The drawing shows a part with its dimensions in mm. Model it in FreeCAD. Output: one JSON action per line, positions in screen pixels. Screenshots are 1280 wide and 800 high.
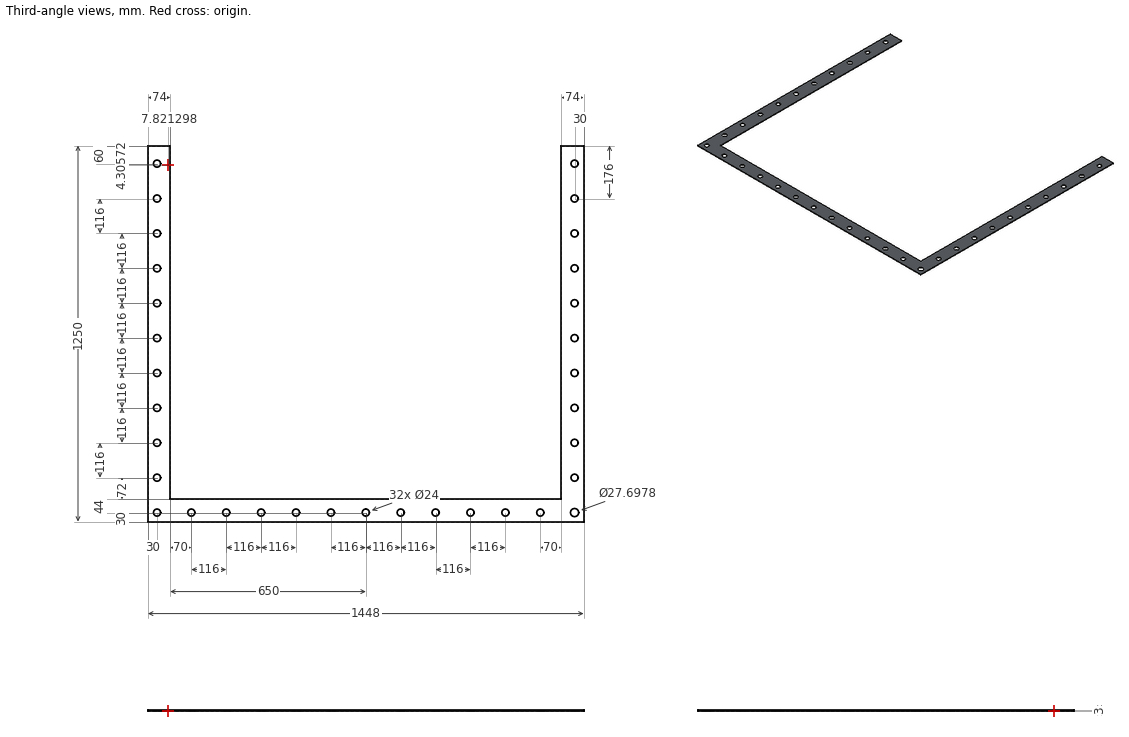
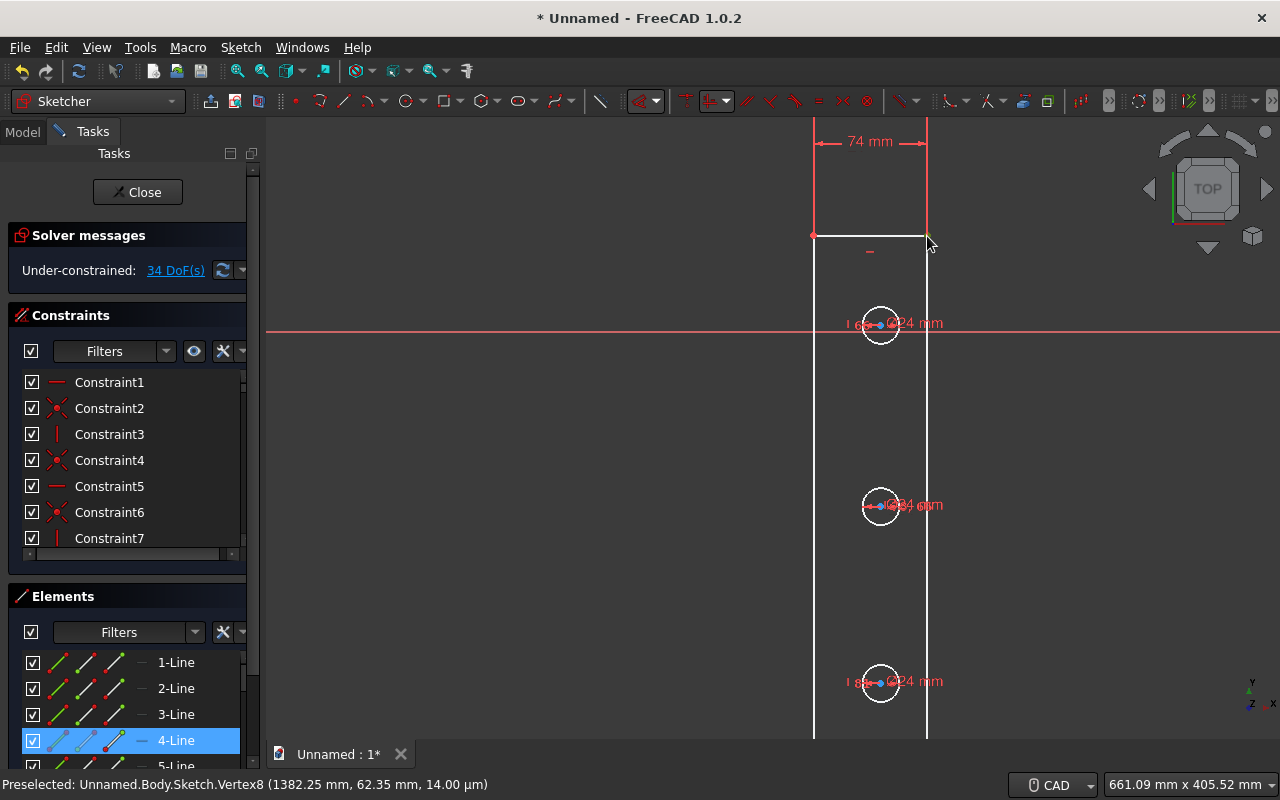
{"action": "left_click", "coordinate": [881, 507]}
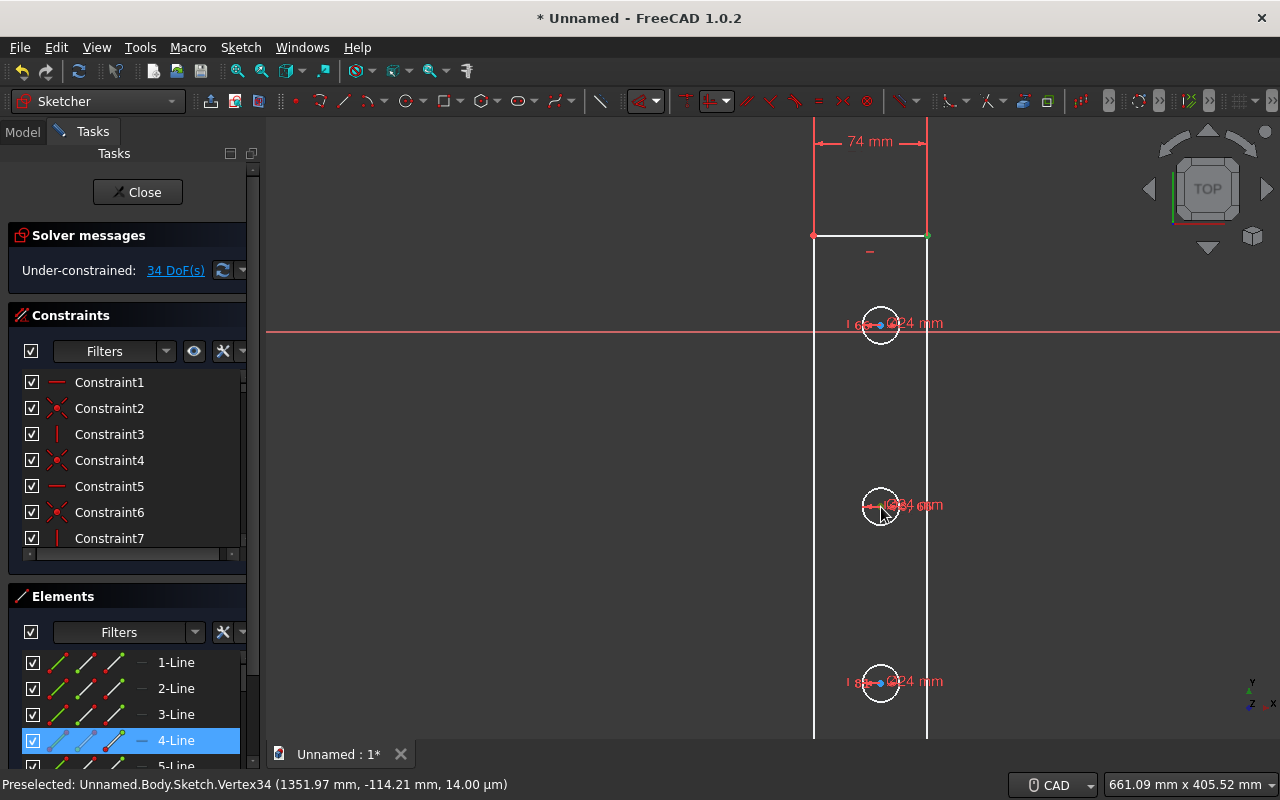
{"action": "key", "text": "l"}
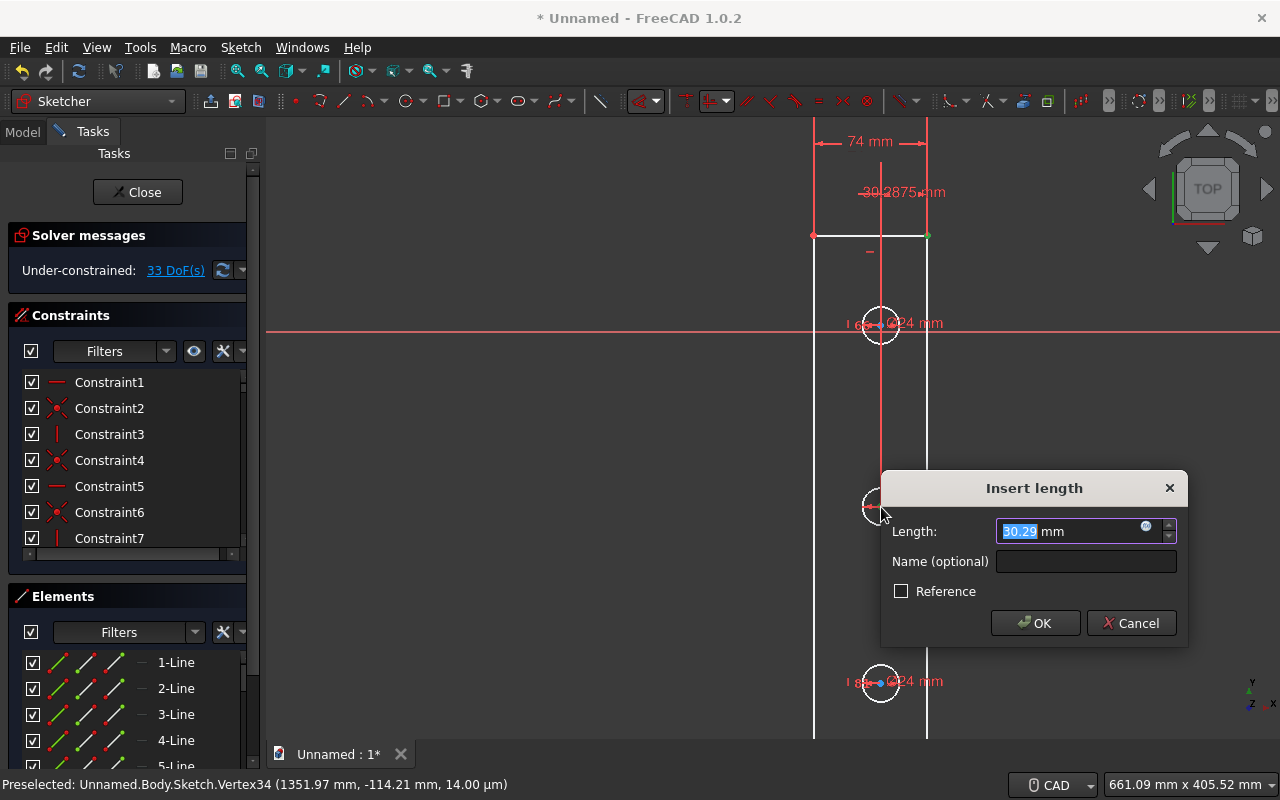
{"action": "type", "text": "30"}
{"action": "key", "text": "Return"}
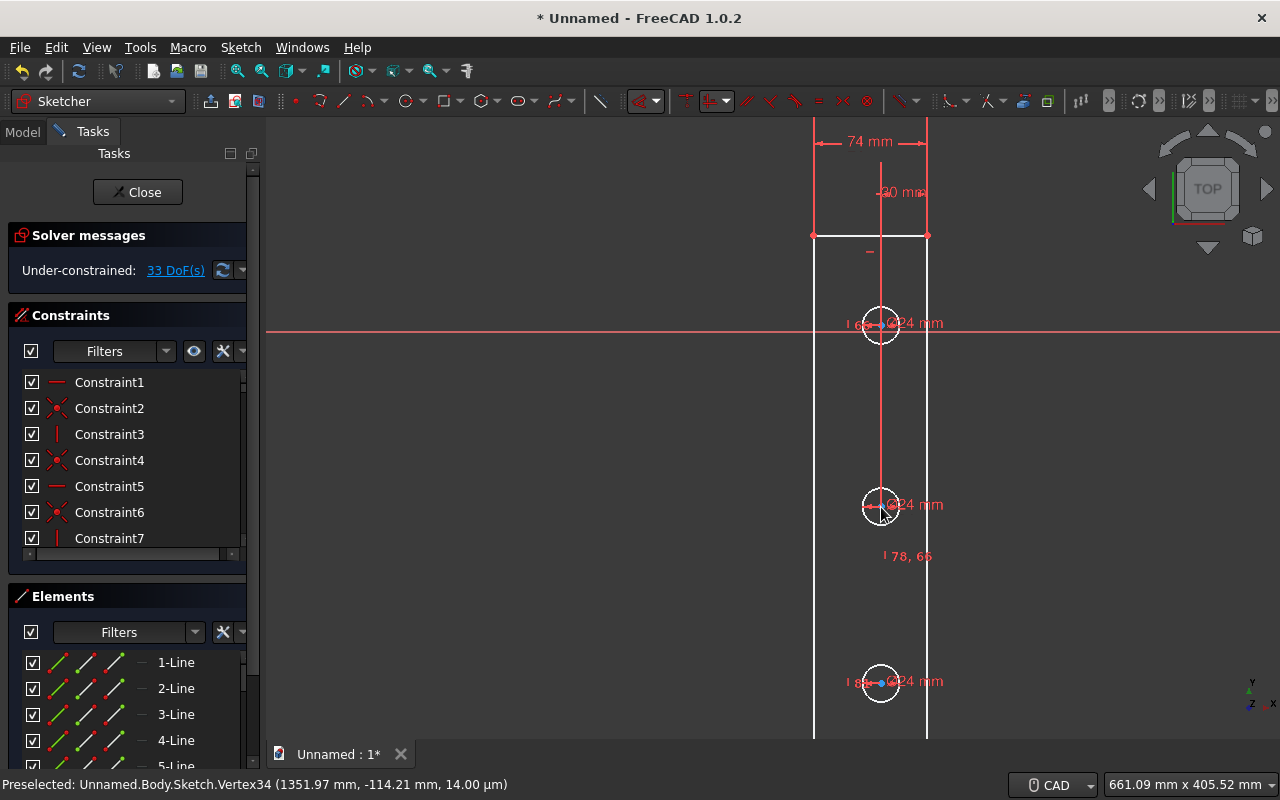
{"action": "left_click", "coordinate": [927, 236]}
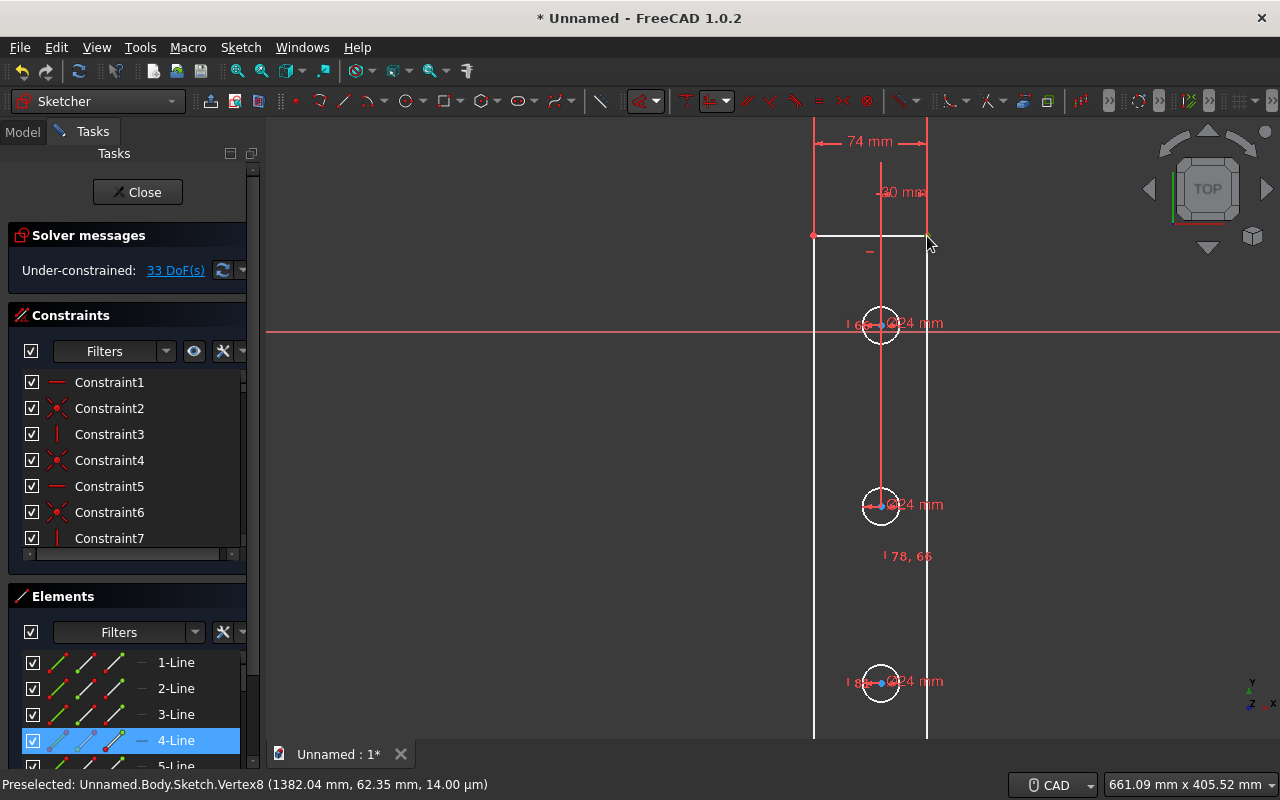
{"action": "left_click", "coordinate": [881, 325]}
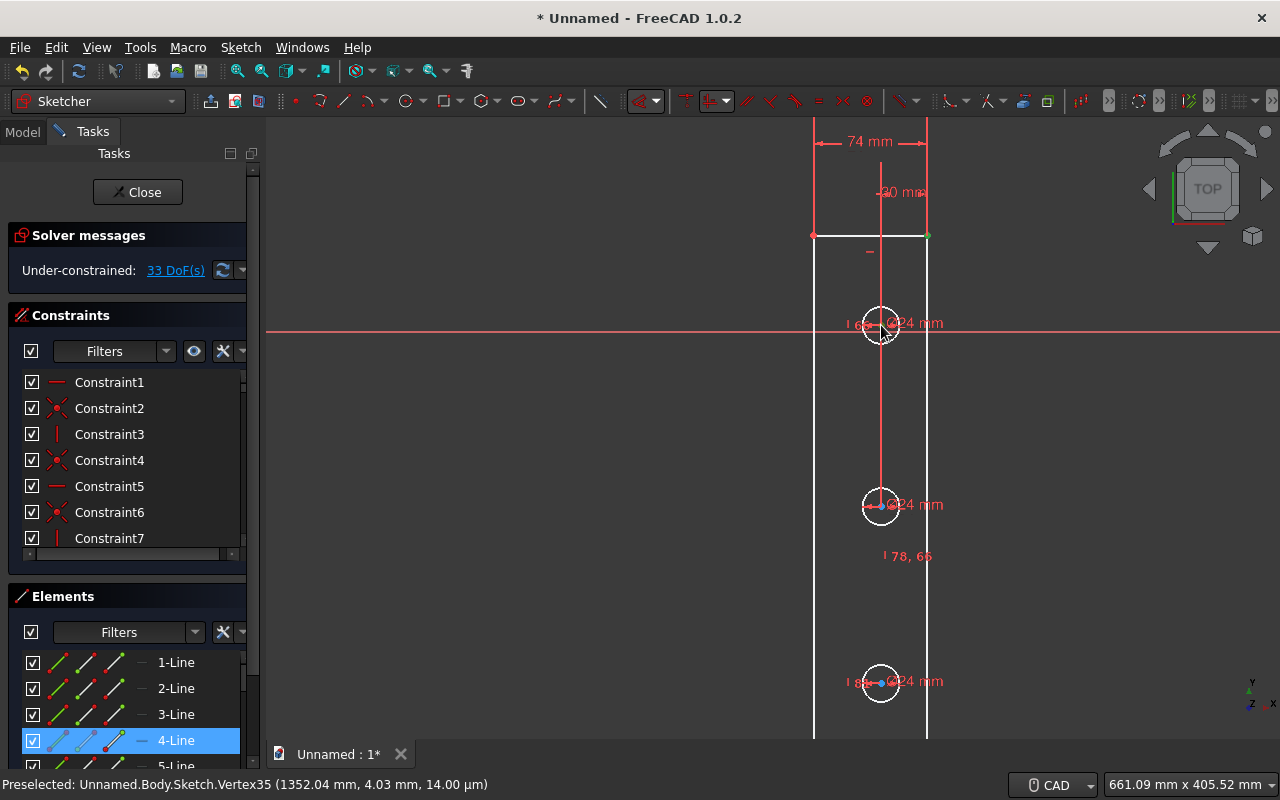
{"action": "key", "text": "i"}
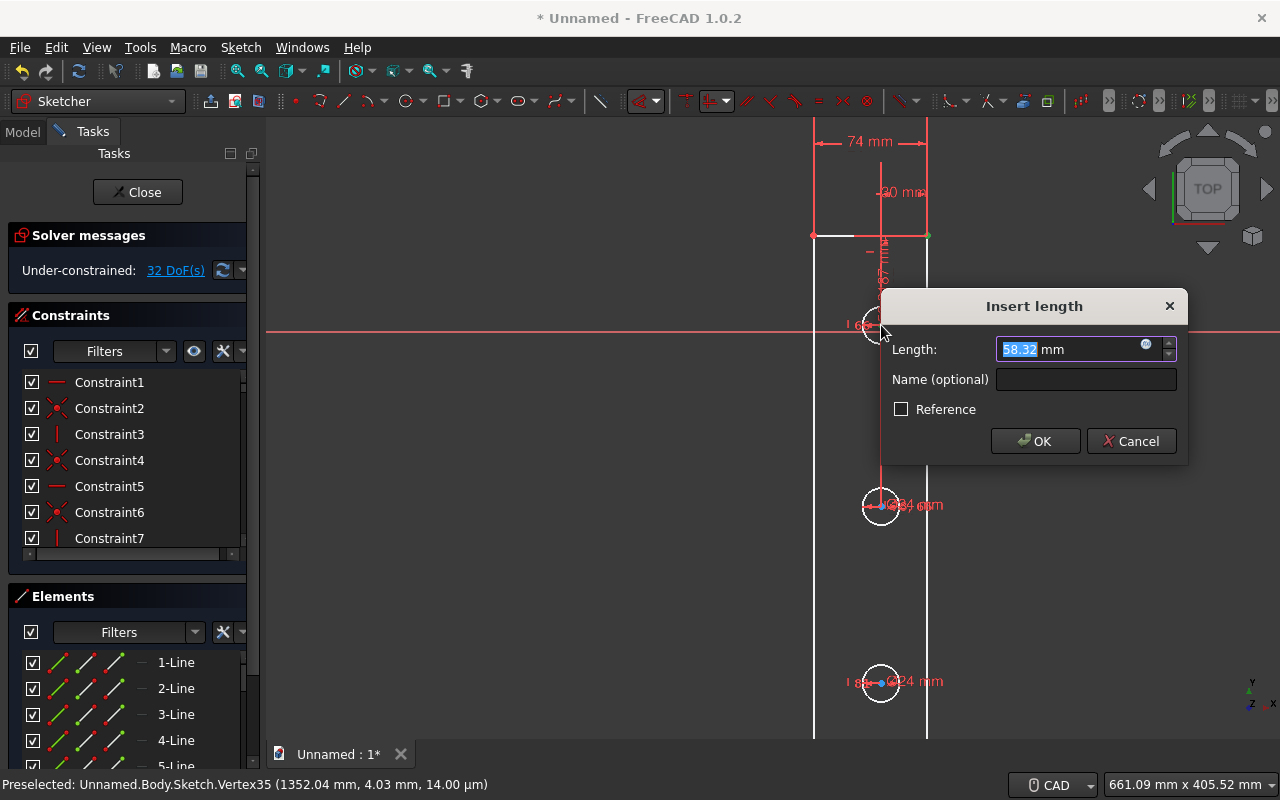
{"action": "type", "text": "60"}
{"action": "key", "text": "Return"}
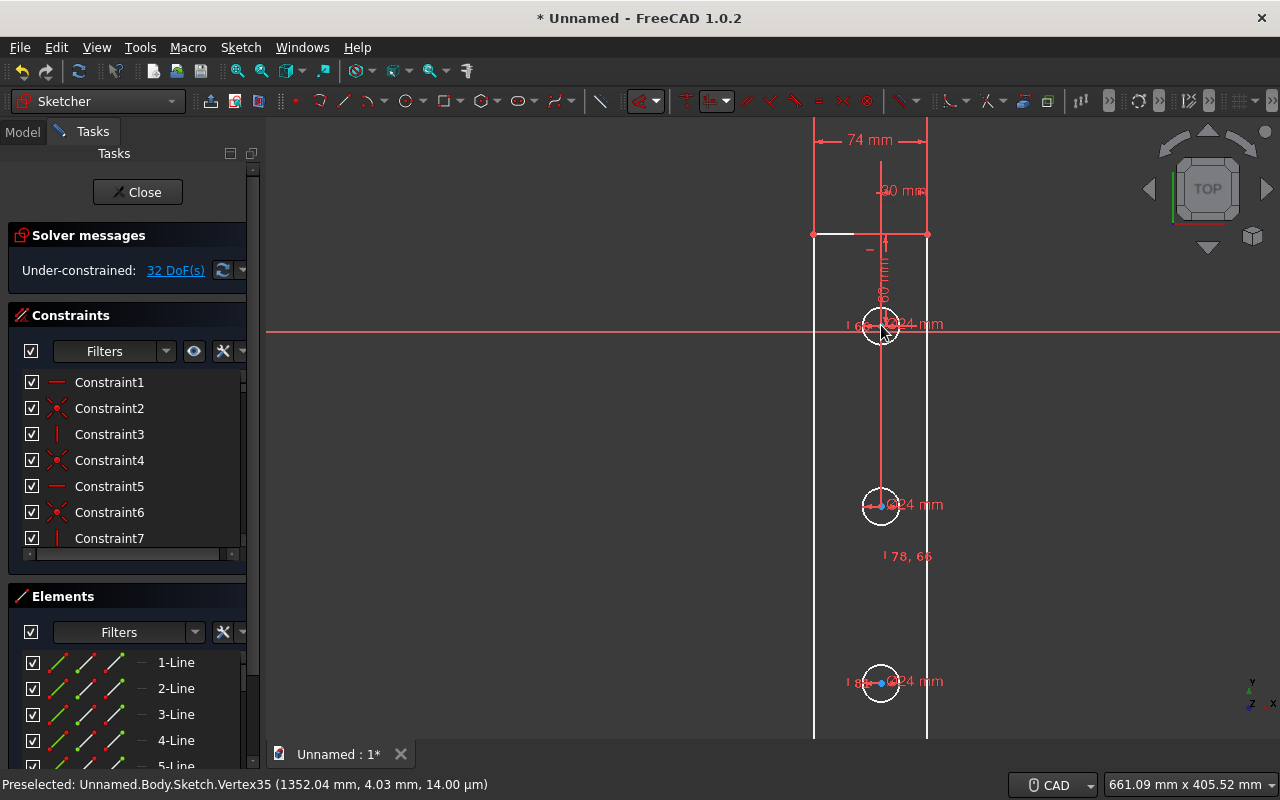
{"action": "scroll", "coordinate": [929, 235], "scroll_direction": "down", "scroll_amount": 8}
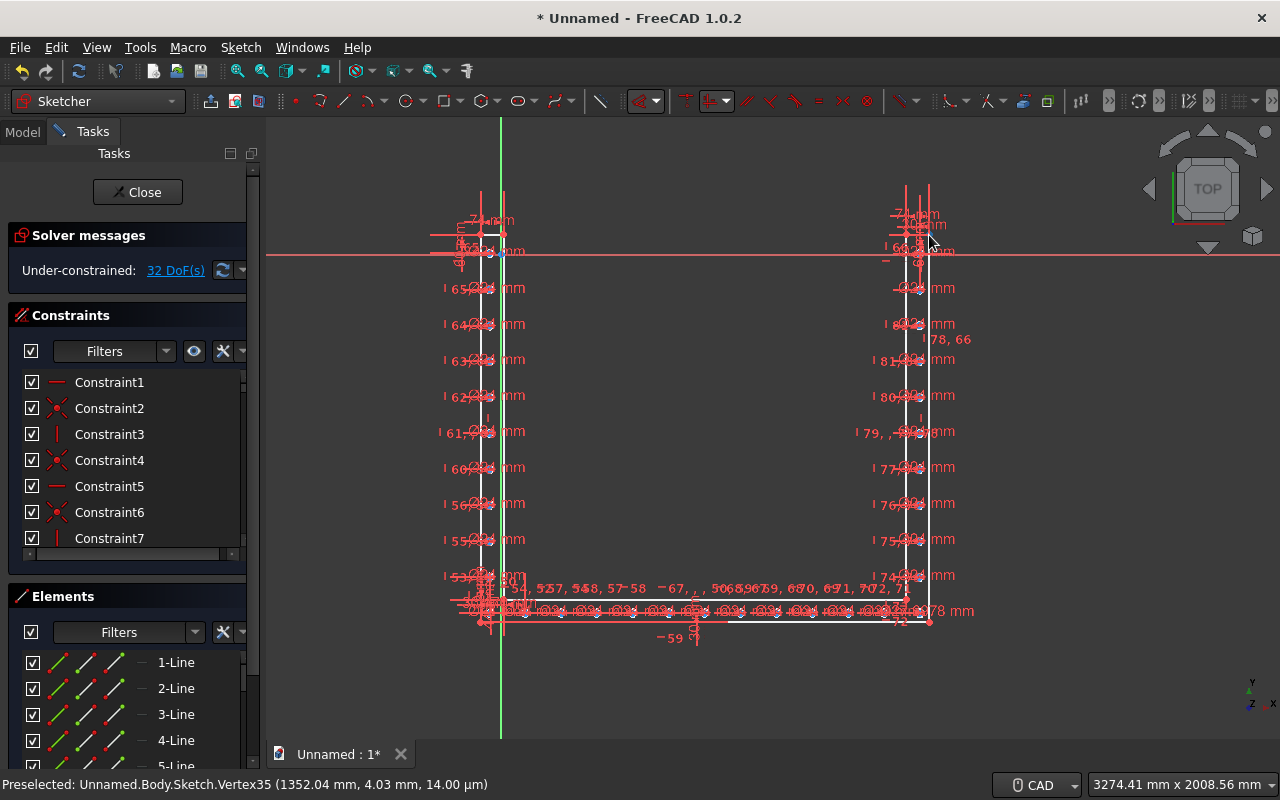
{"action": "scroll", "coordinate": [906, 600], "scroll_direction": "up", "scroll_amount": 4}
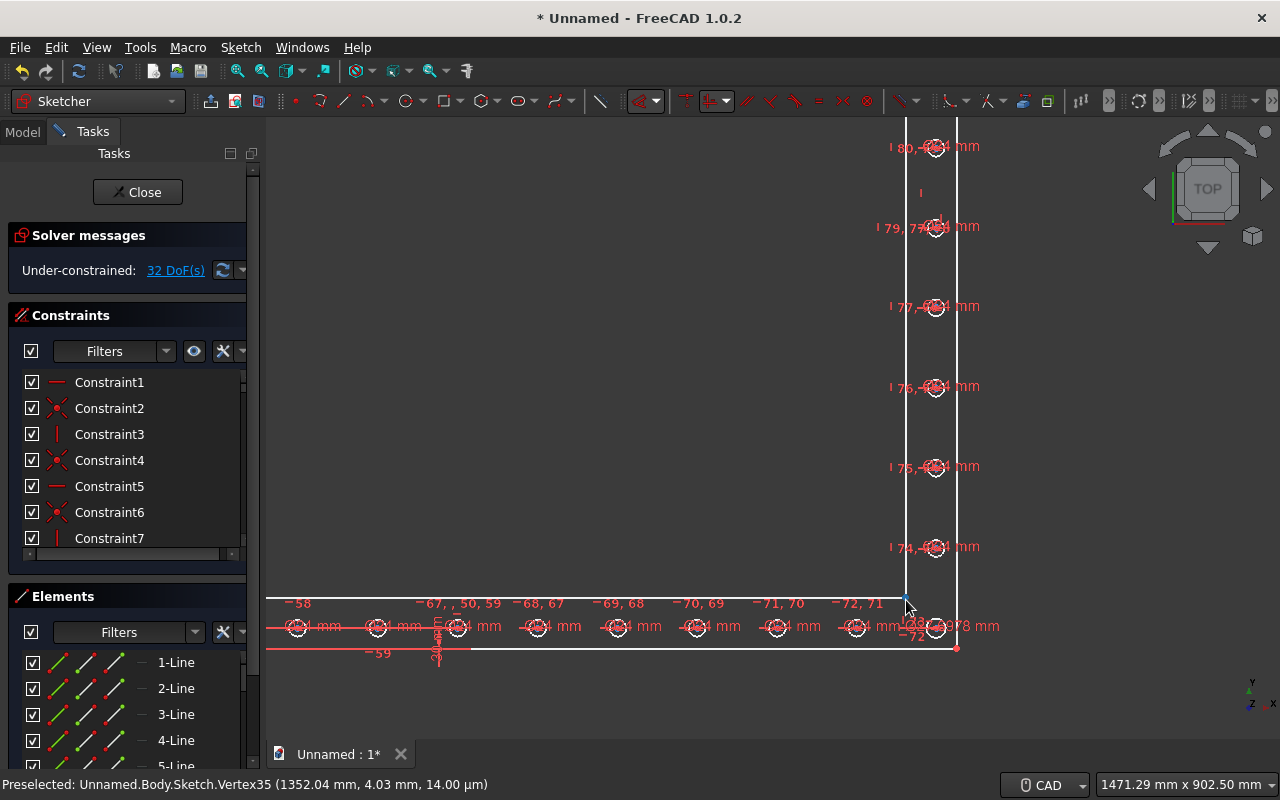
{"action": "left_click", "coordinate": [906, 598]}